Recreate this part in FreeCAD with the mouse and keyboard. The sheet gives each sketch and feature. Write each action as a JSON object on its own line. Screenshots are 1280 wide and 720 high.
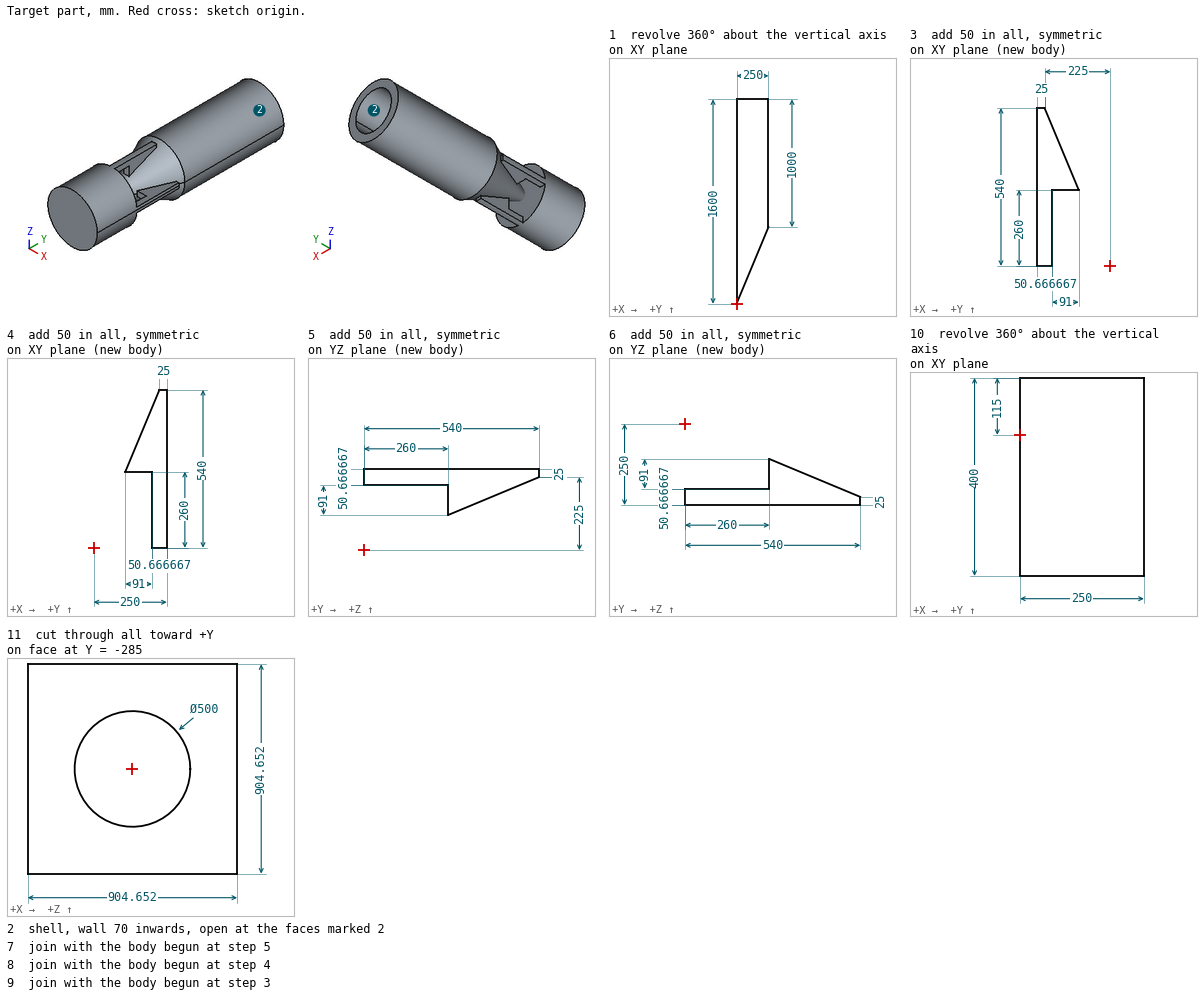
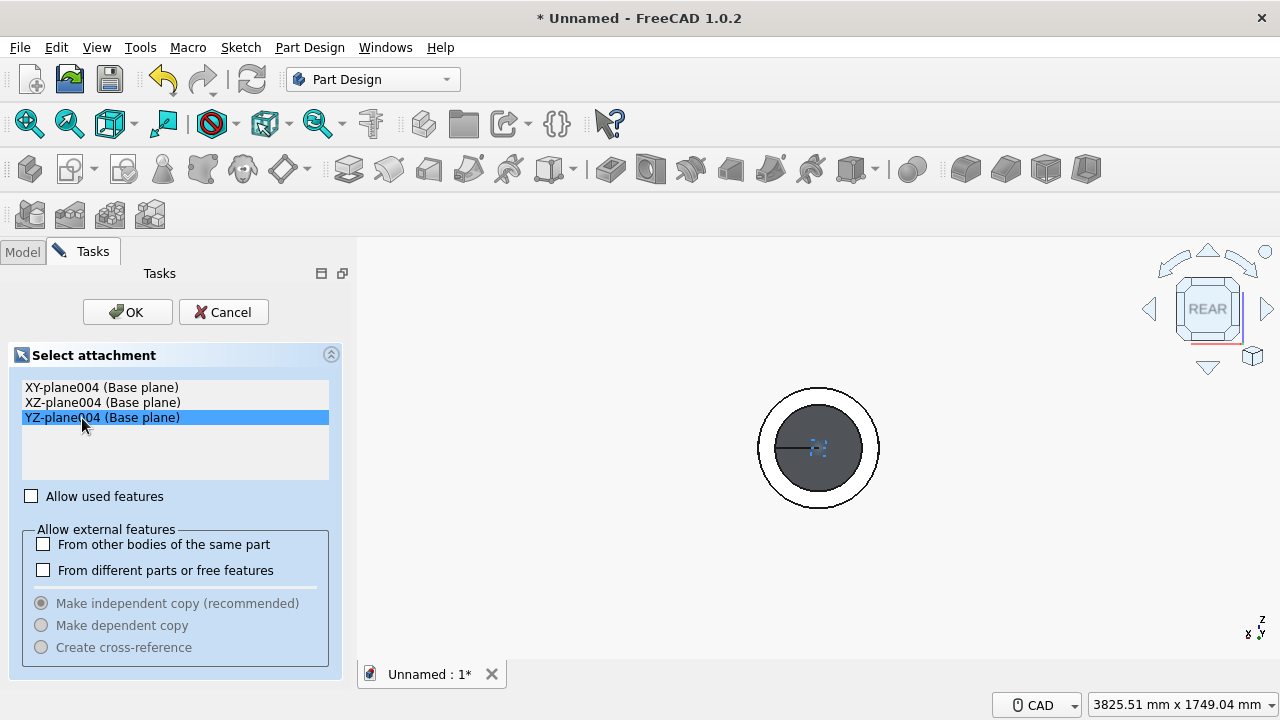
{"action": "left_click", "coordinate": [128, 312]}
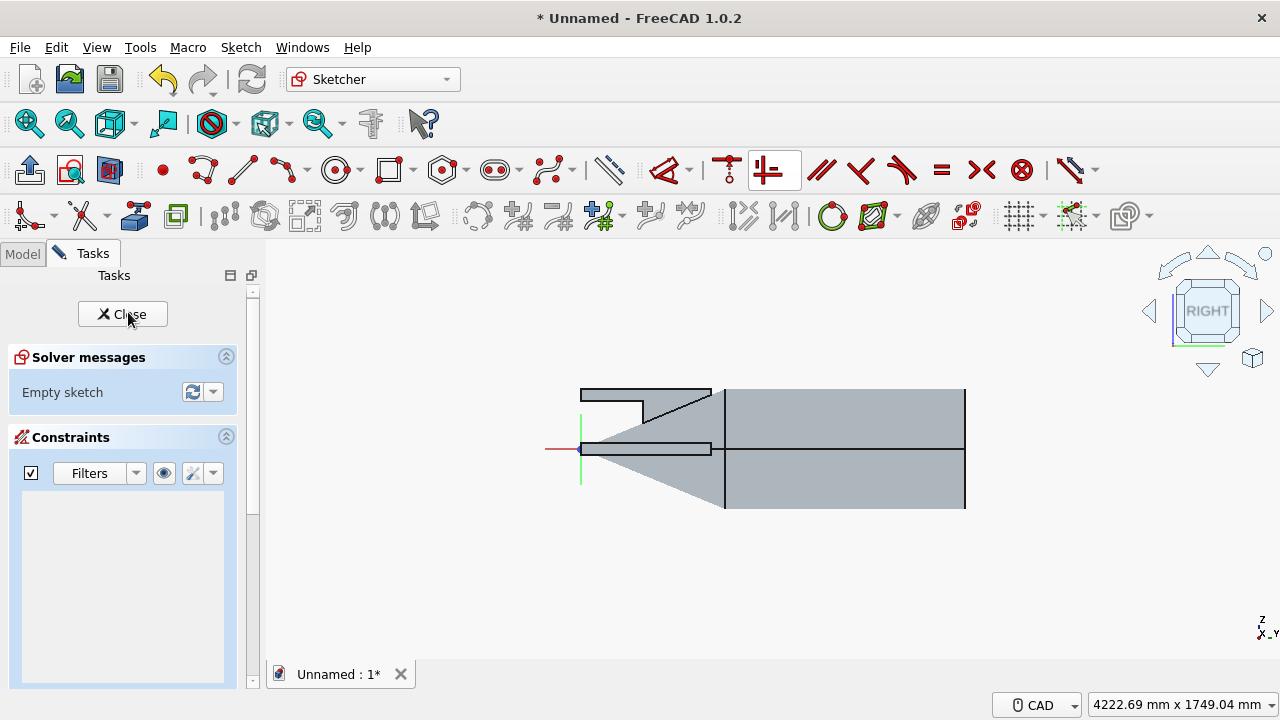
{"action": "scroll", "coordinate": [626, 489], "scroll_direction": "up", "scroll_amount": 7}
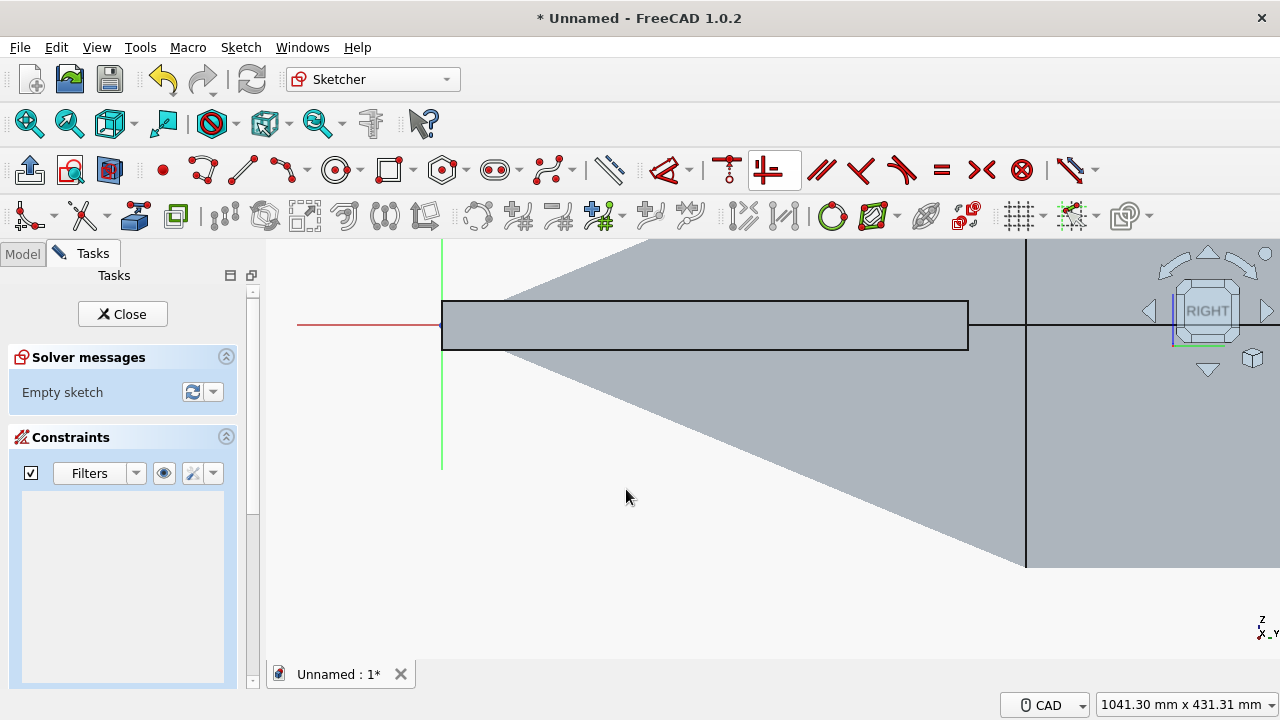
{"action": "left_click", "coordinate": [204, 170]}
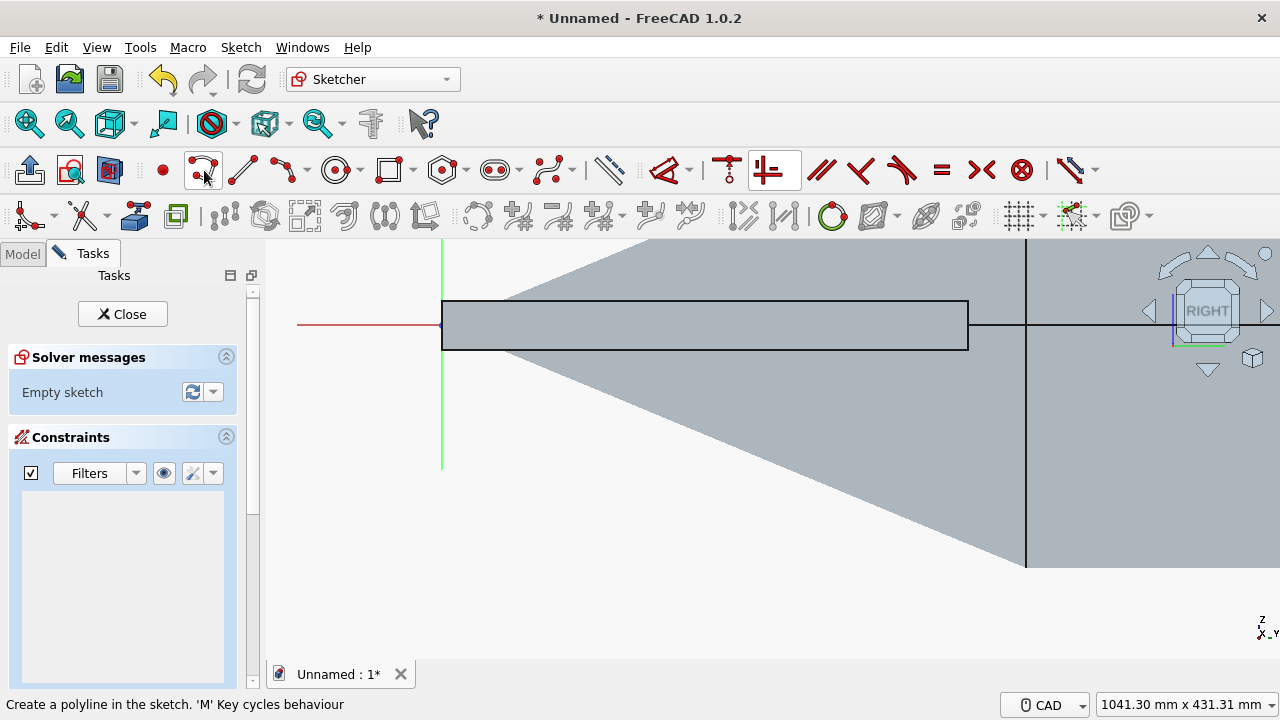
{"action": "left_click", "coordinate": [442, 519]}
{"action": "left_click", "coordinate": [451, 569]}
{"action": "left_click", "coordinate": [968, 569]}
{"action": "left_click", "coordinate": [968, 544]}
{"action": "left_click", "coordinate": [695, 431]}
{"action": "left_click", "coordinate": [695, 519]}
{"action": "left_click", "coordinate": [442, 520]}
{"action": "key", "text": "Escape"}
{"action": "key", "text": "Escape"}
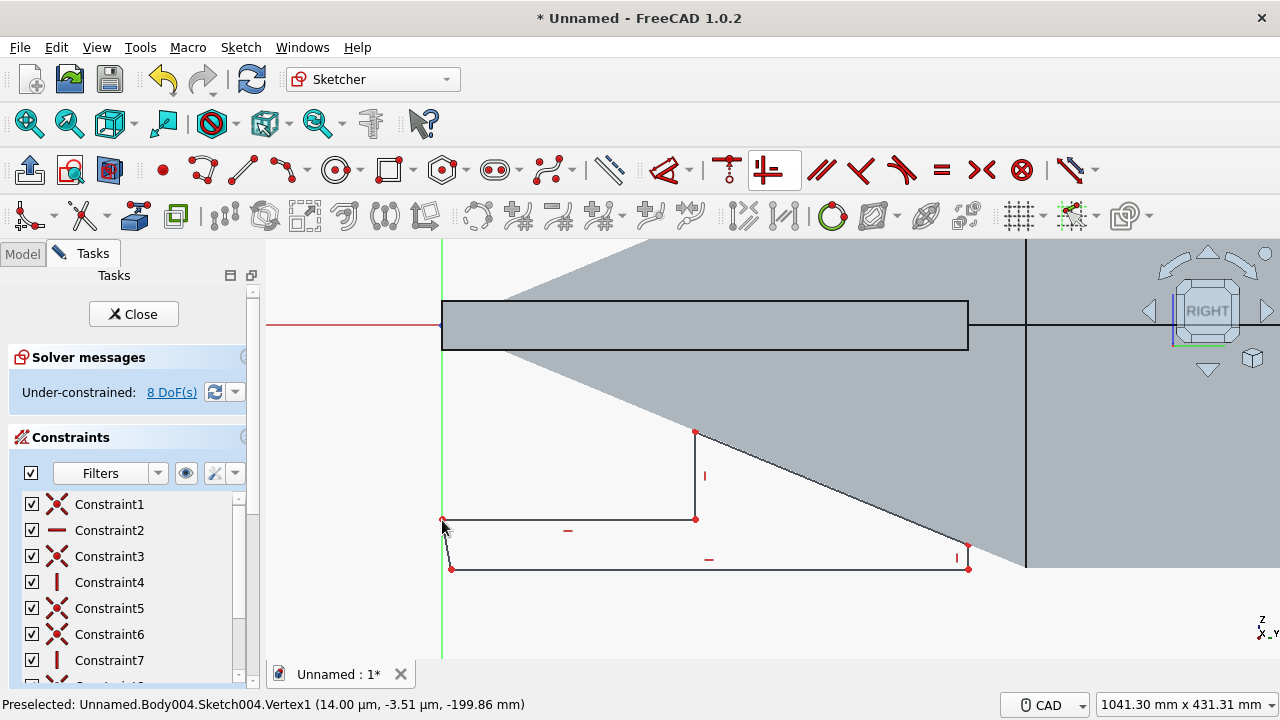
{"action": "left_click", "coordinate": [445, 535]}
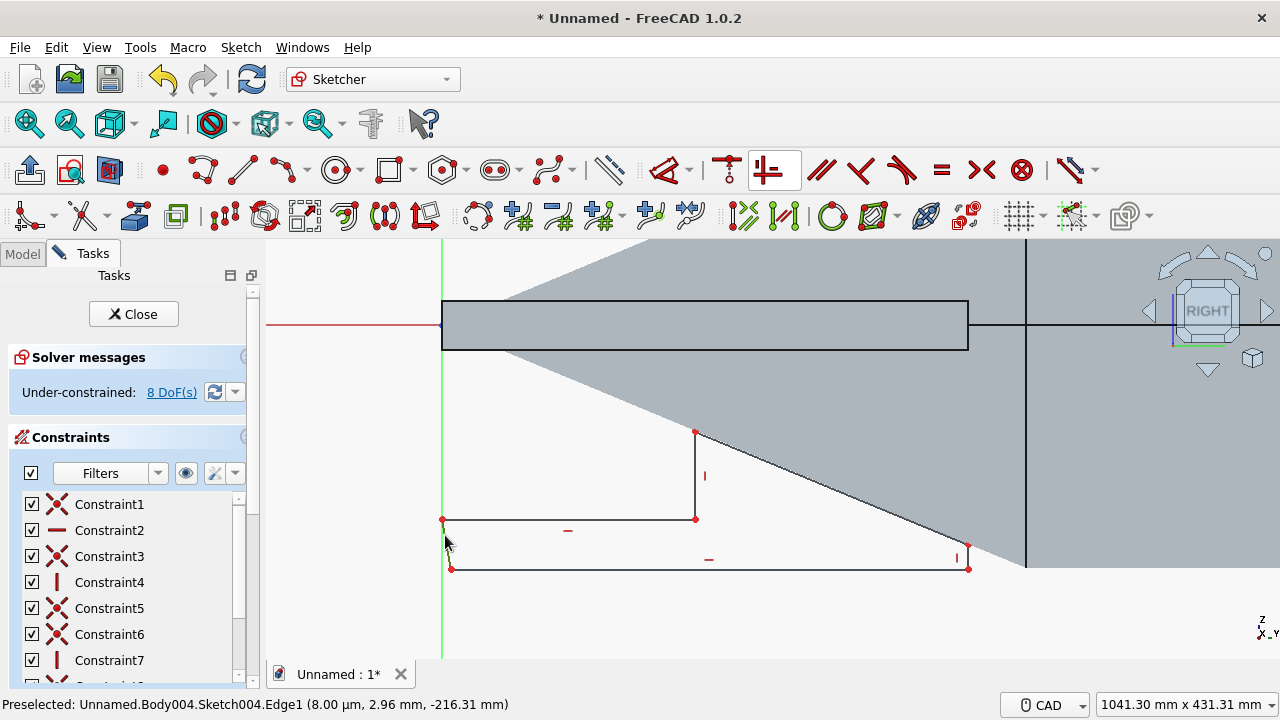
{"action": "key", "text": "v"}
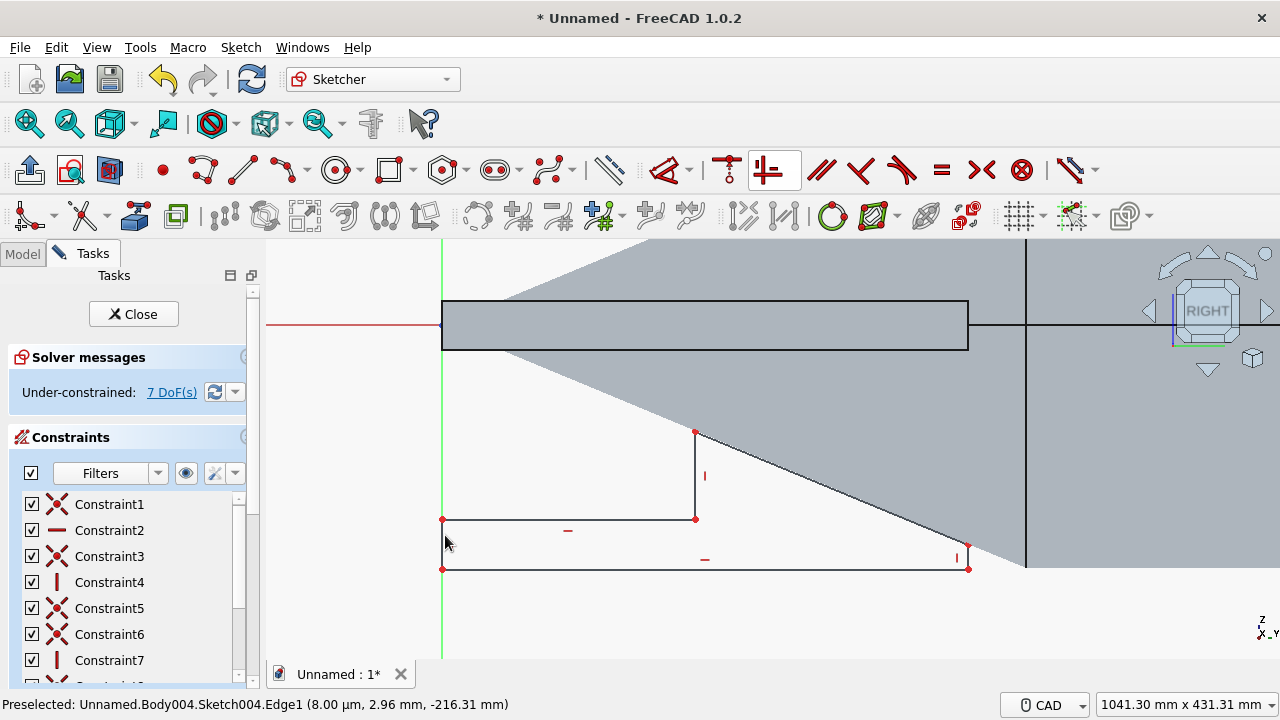
{"action": "left_click", "coordinate": [442, 520]}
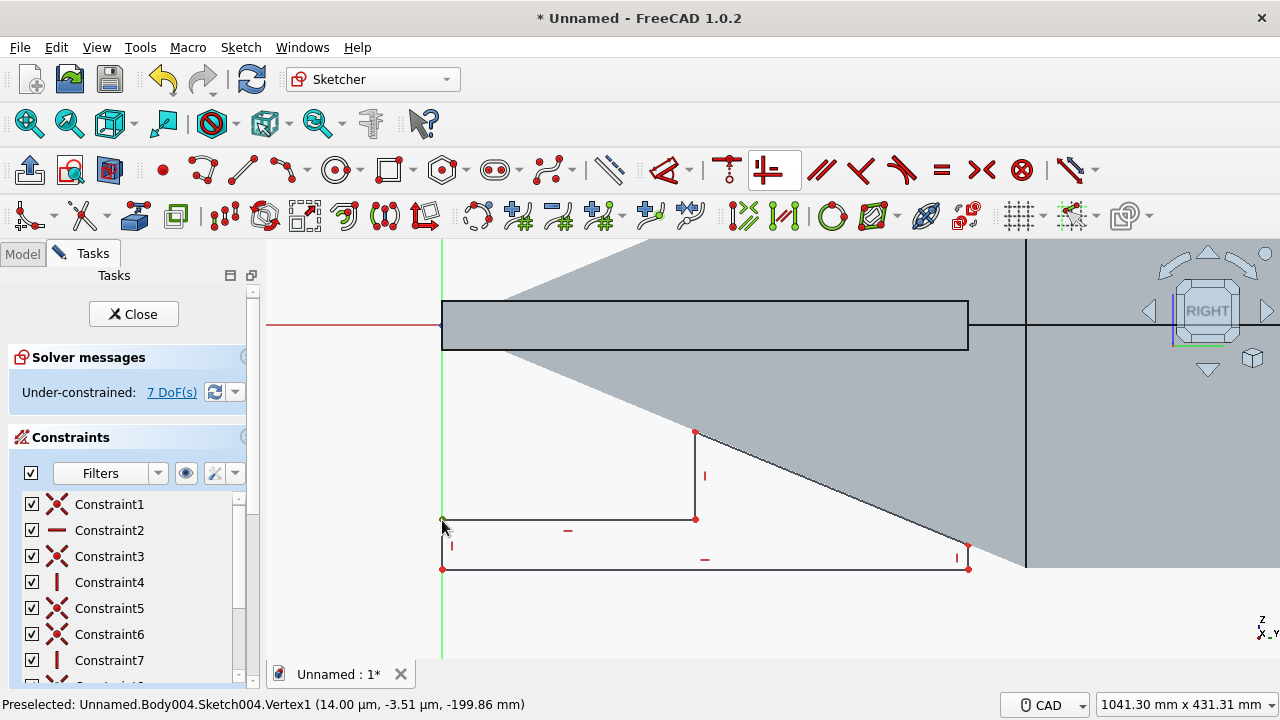
{"action": "left_click", "coordinate": [442, 605]}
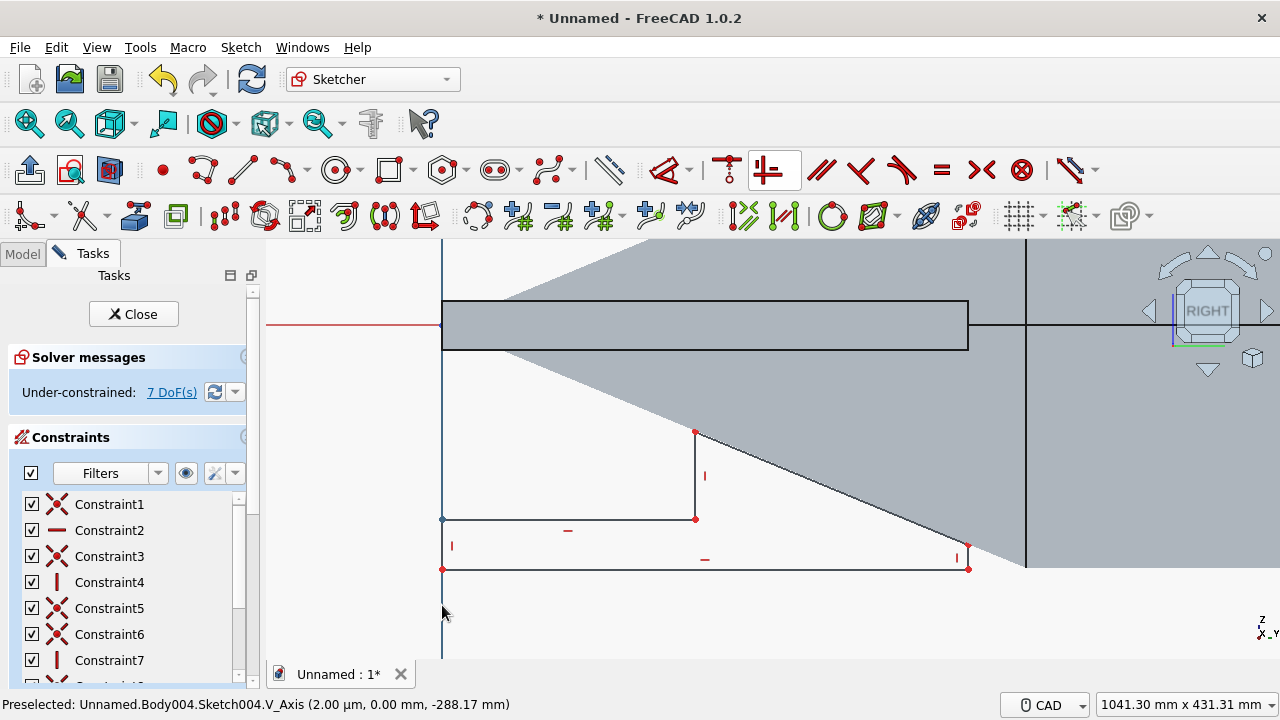
{"action": "left_click", "coordinate": [728, 170]}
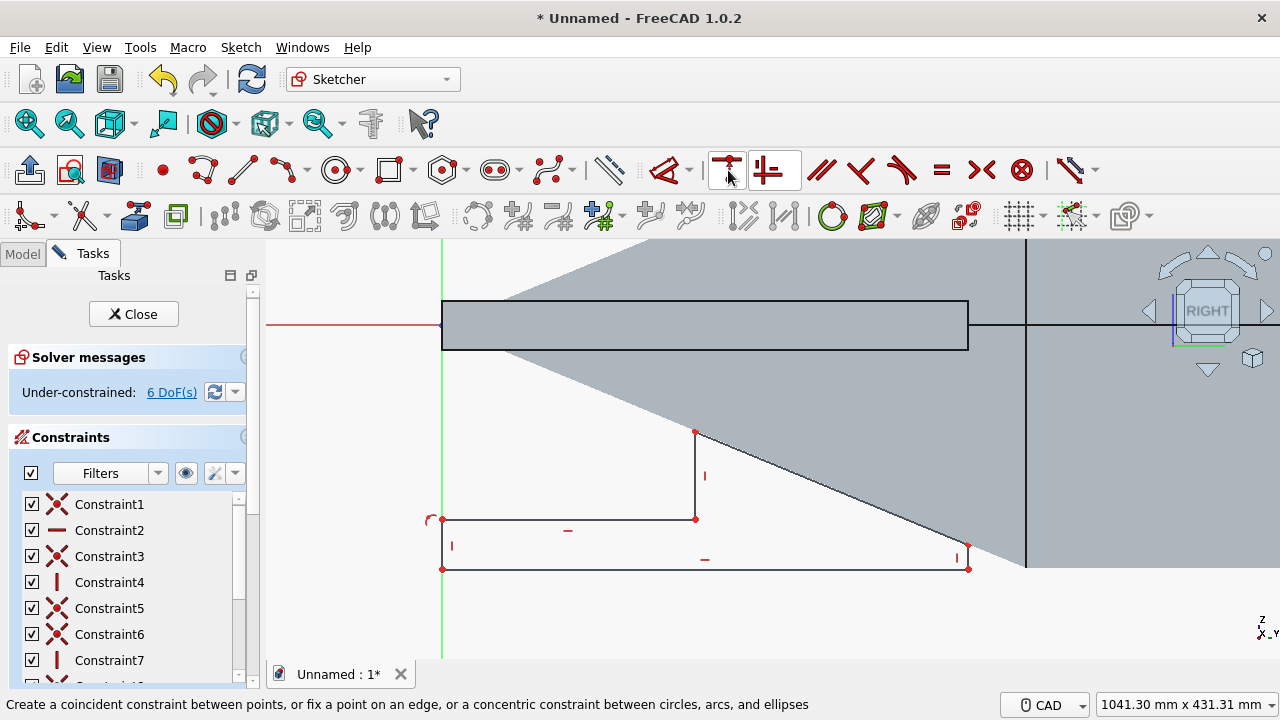
{"action": "left_click", "coordinate": [664, 170]}